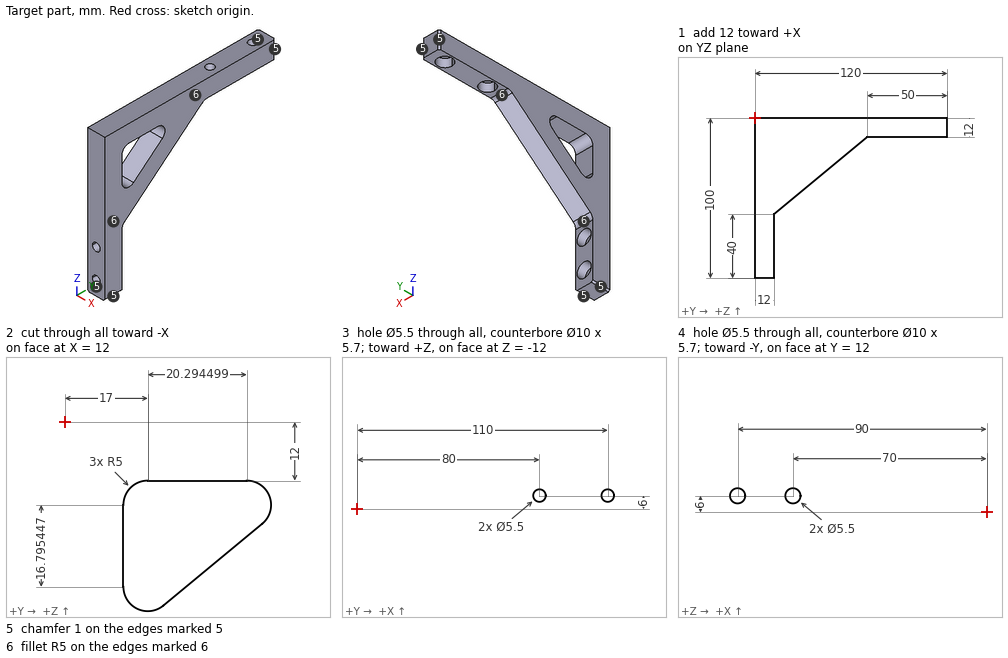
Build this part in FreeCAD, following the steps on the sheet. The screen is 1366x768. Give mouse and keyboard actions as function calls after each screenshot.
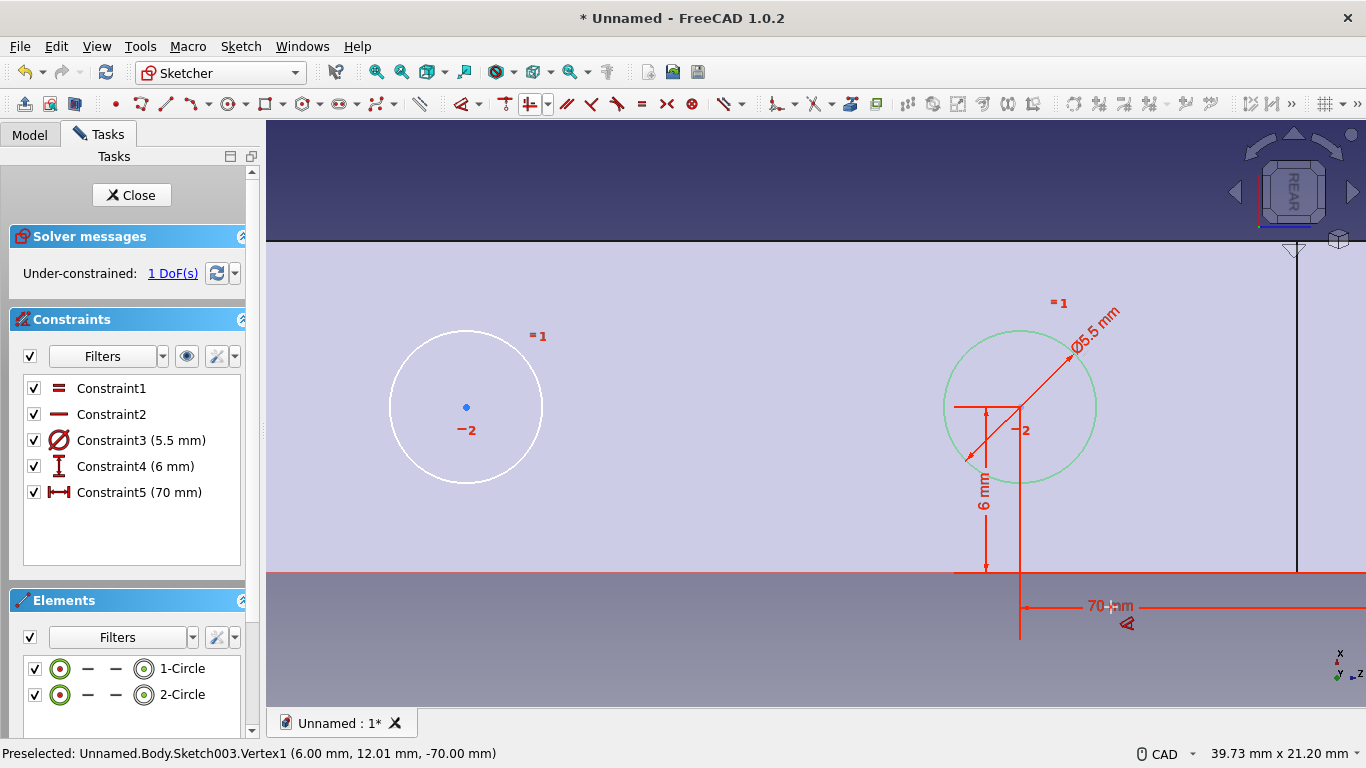
click(466, 407)
click(834, 607)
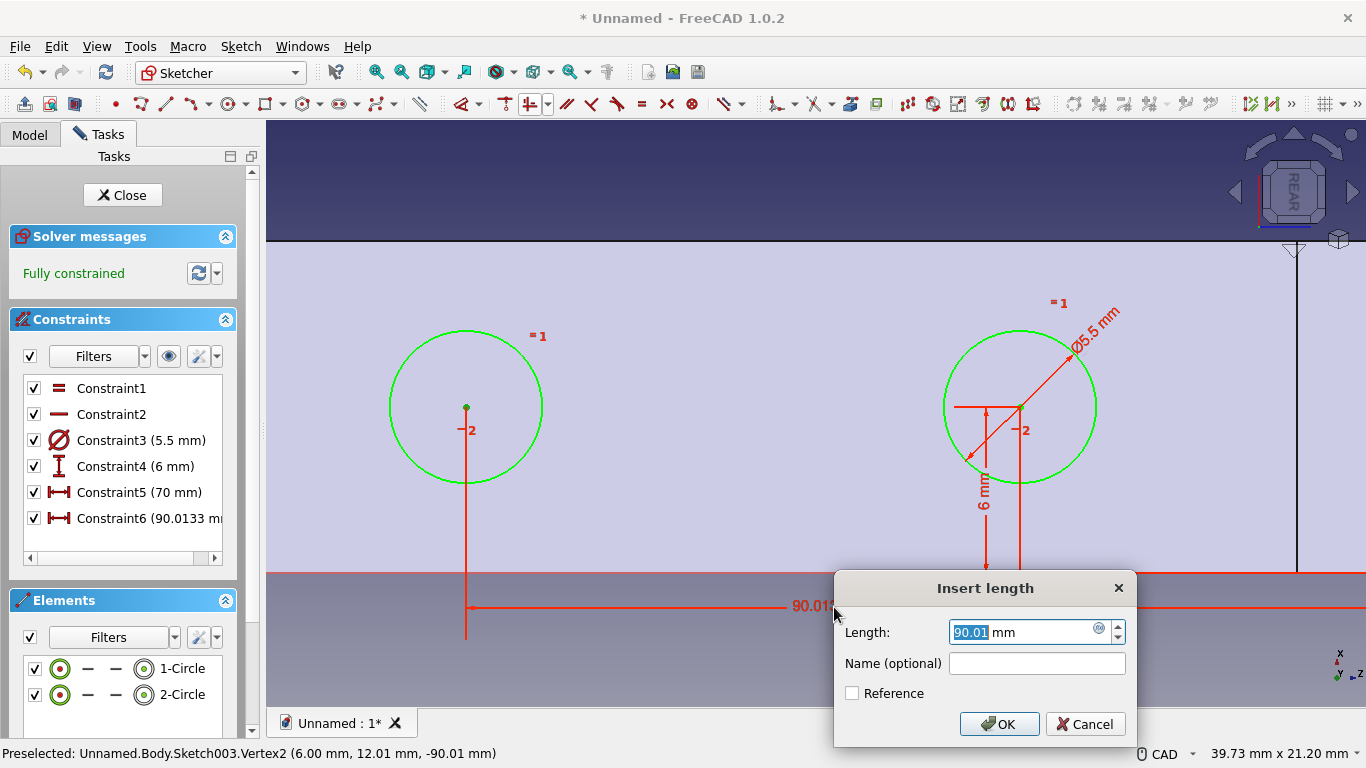
text(90)
key(Return)
key(Escape)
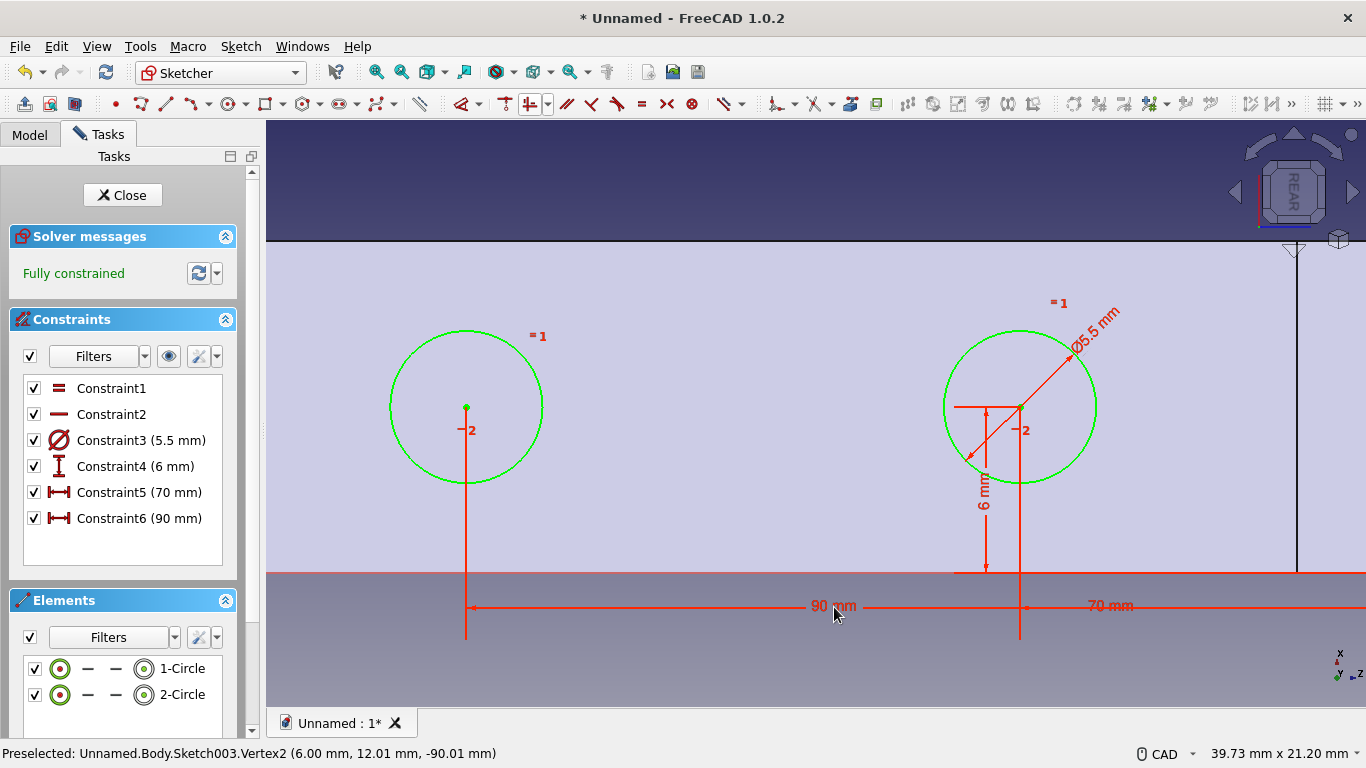
click(123, 195)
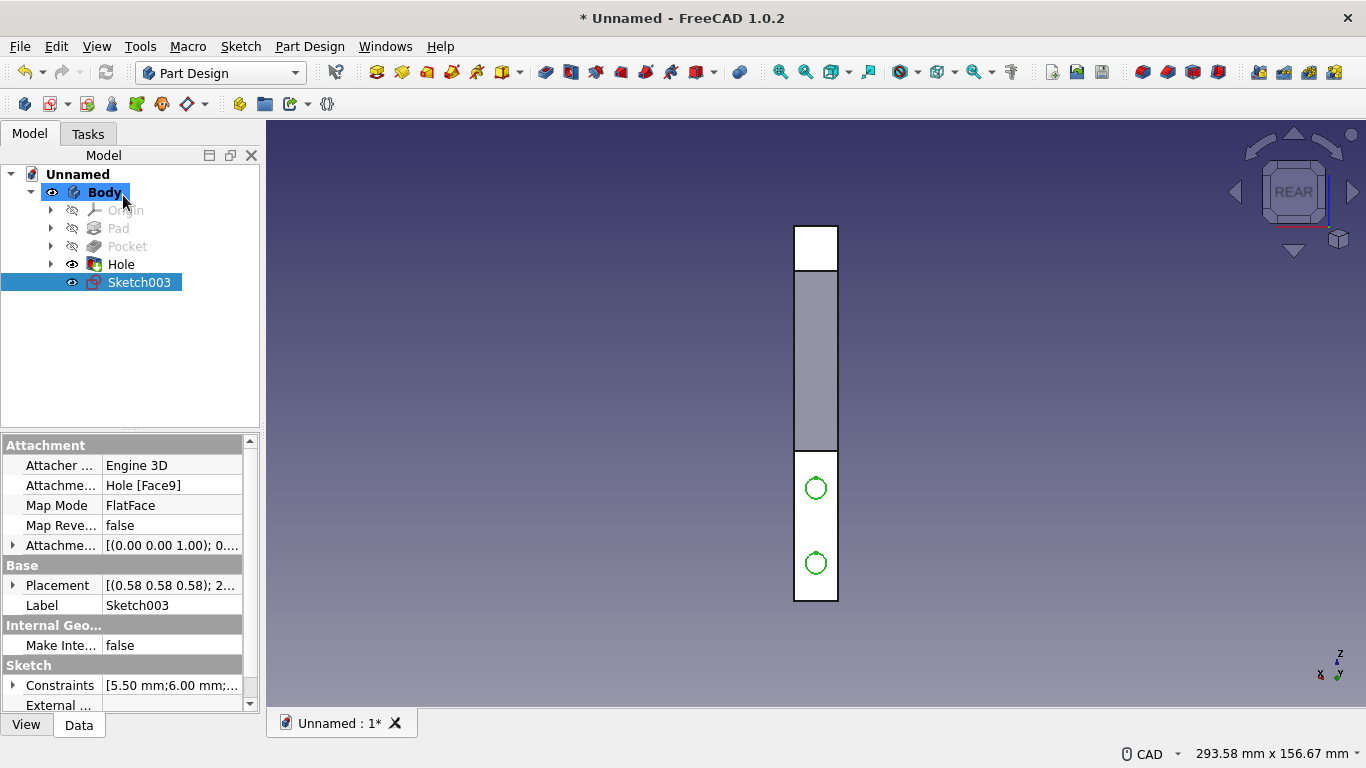
click(571, 72)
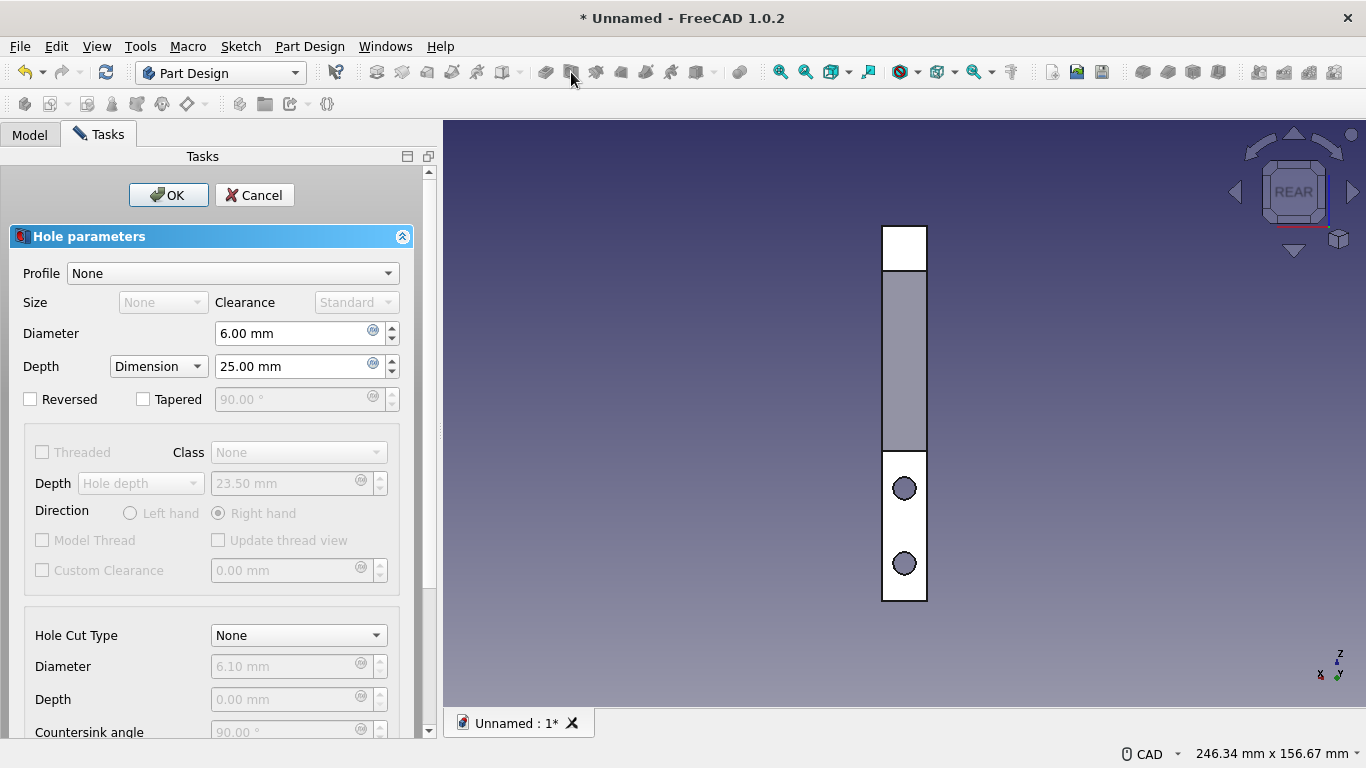
triple_click(300, 334)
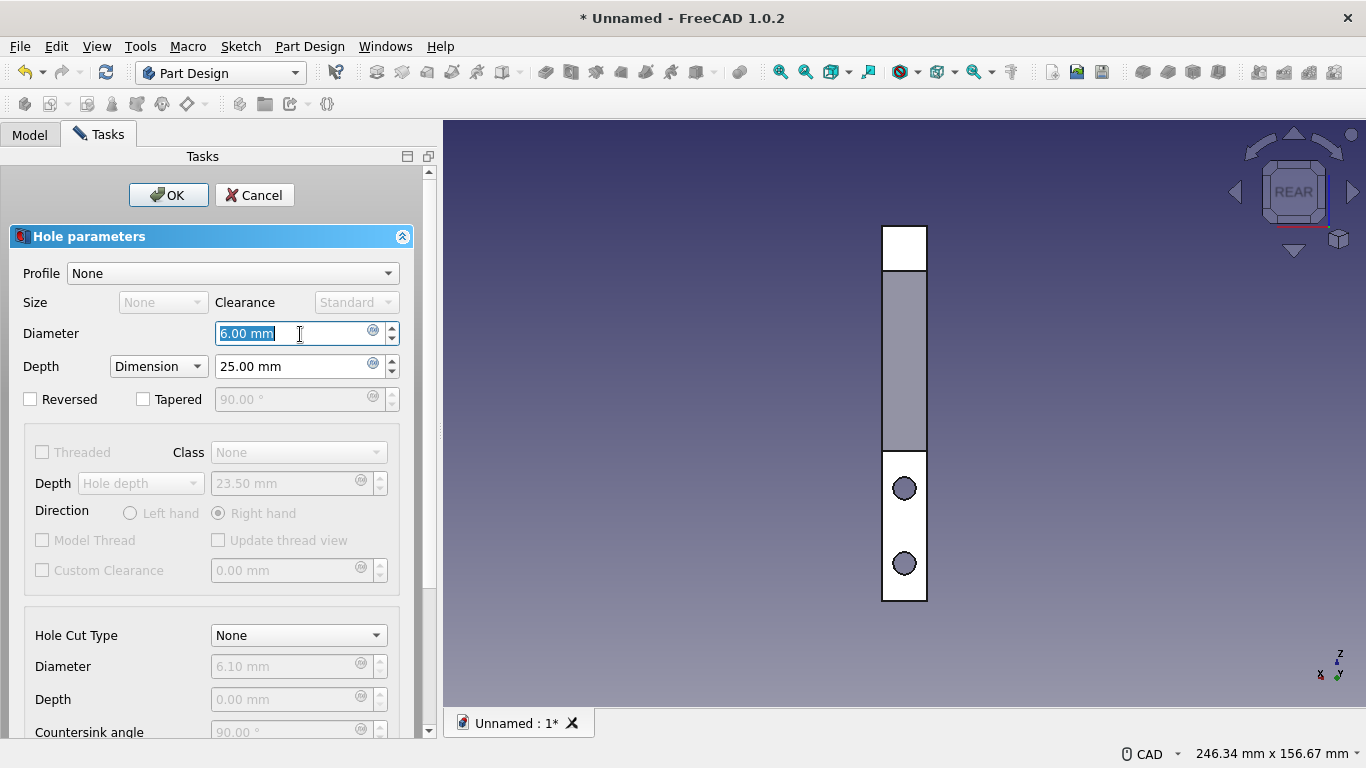
text(5.5)
key(Tab)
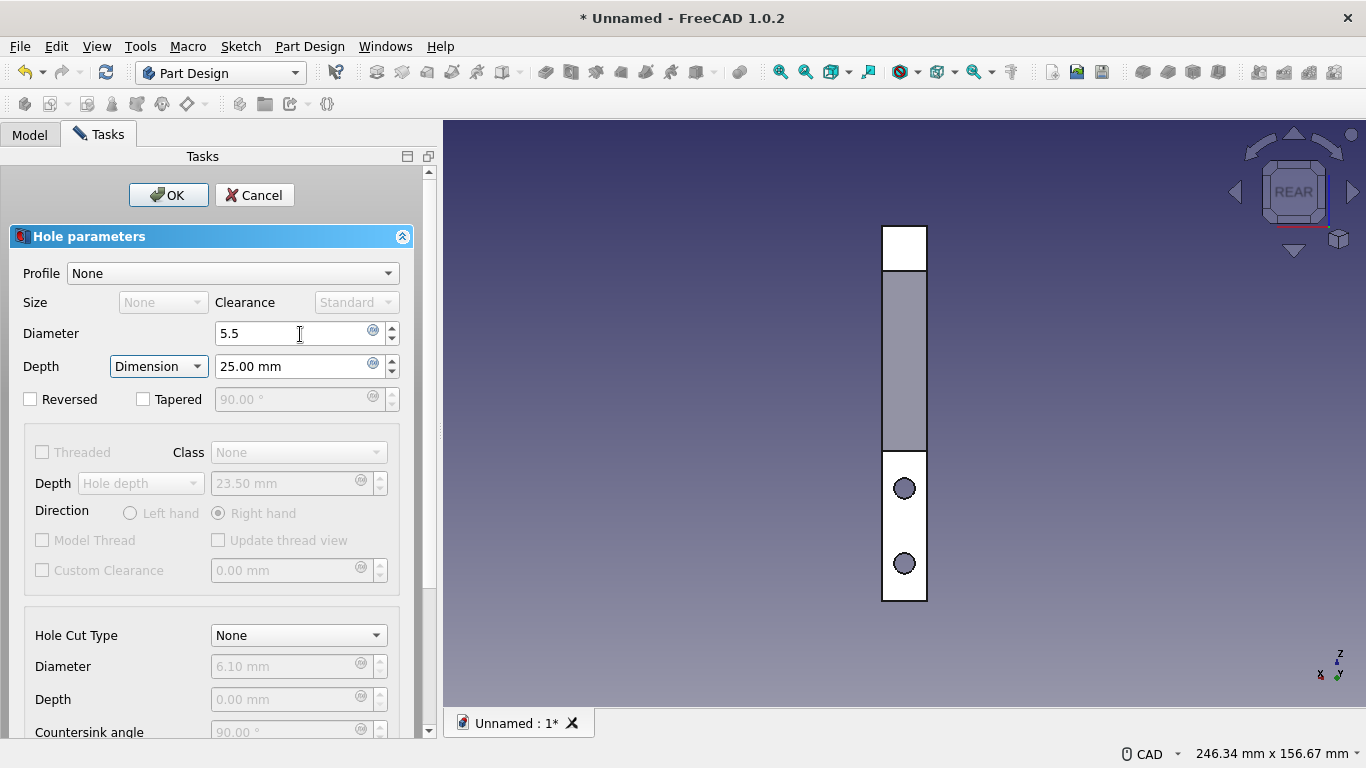
click(160, 366)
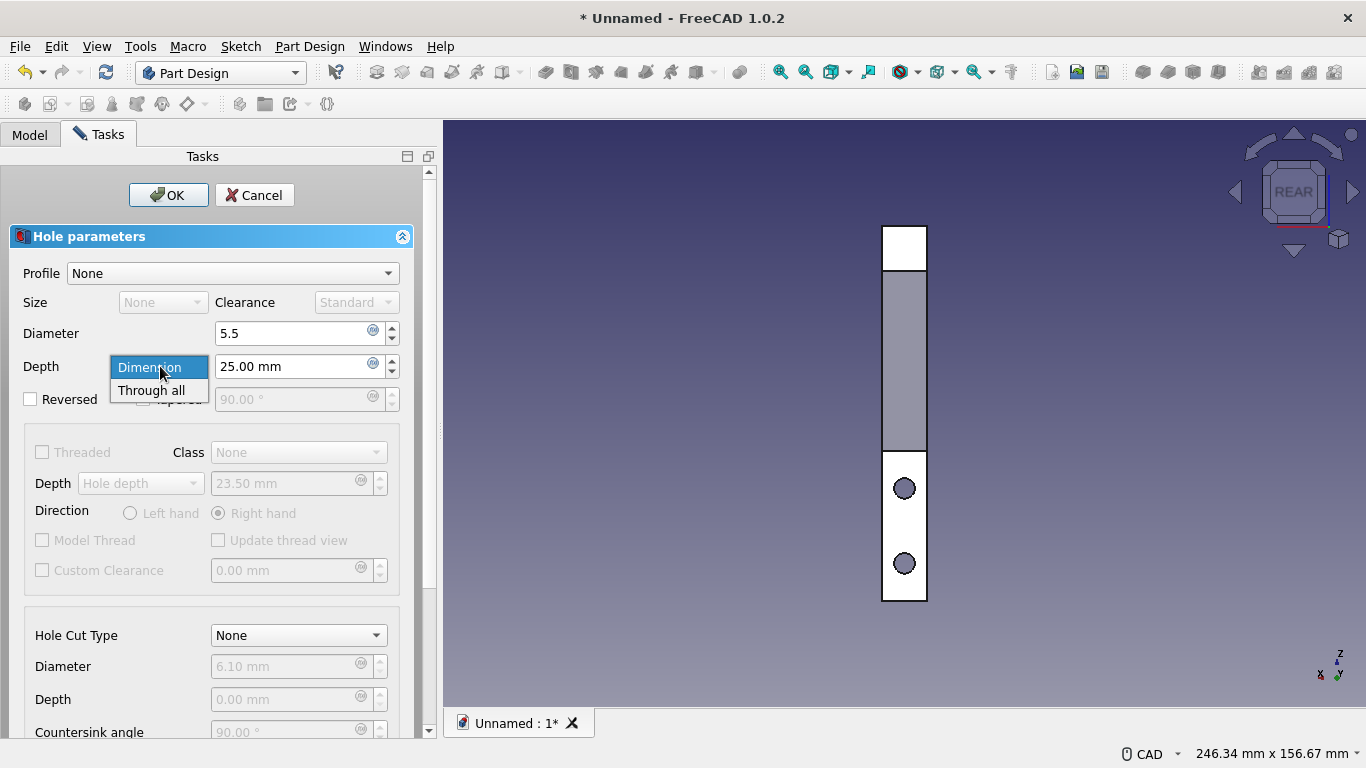
click(158, 390)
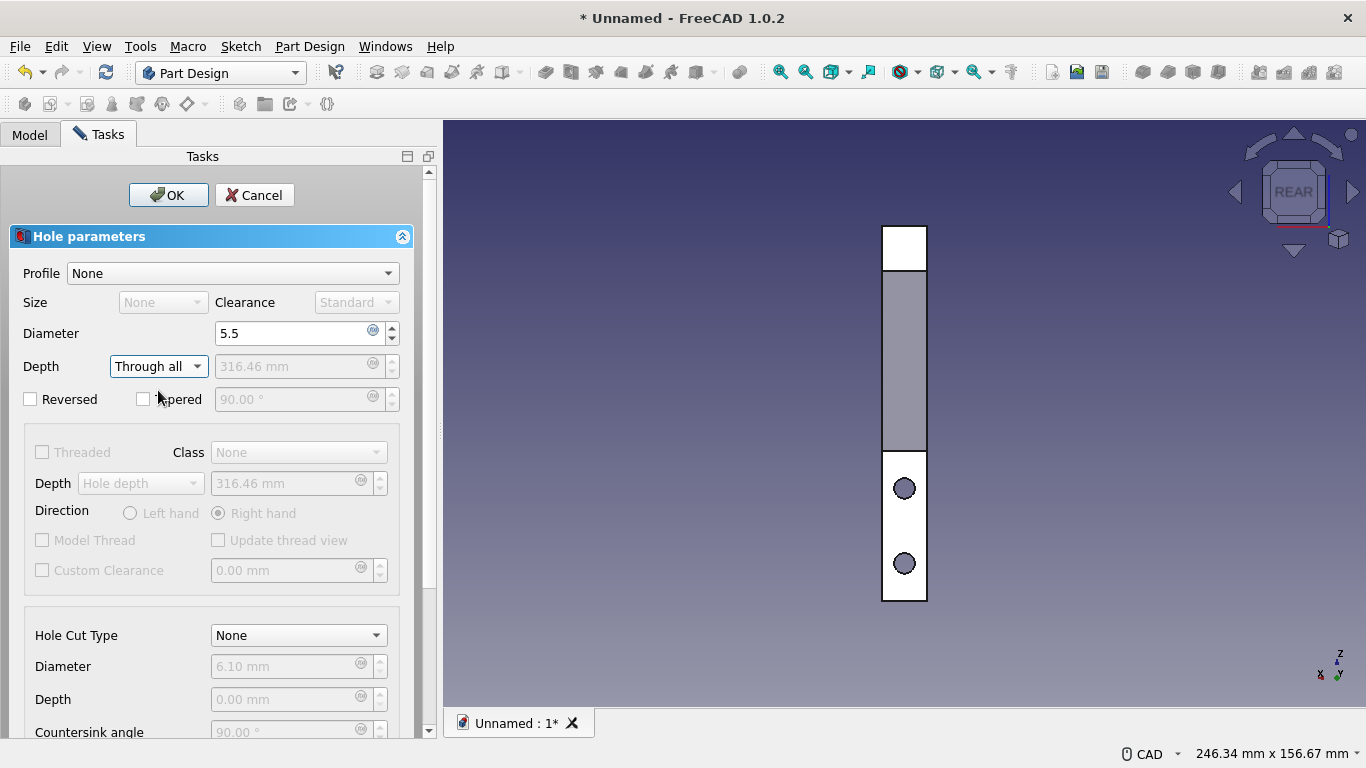
click(300, 636)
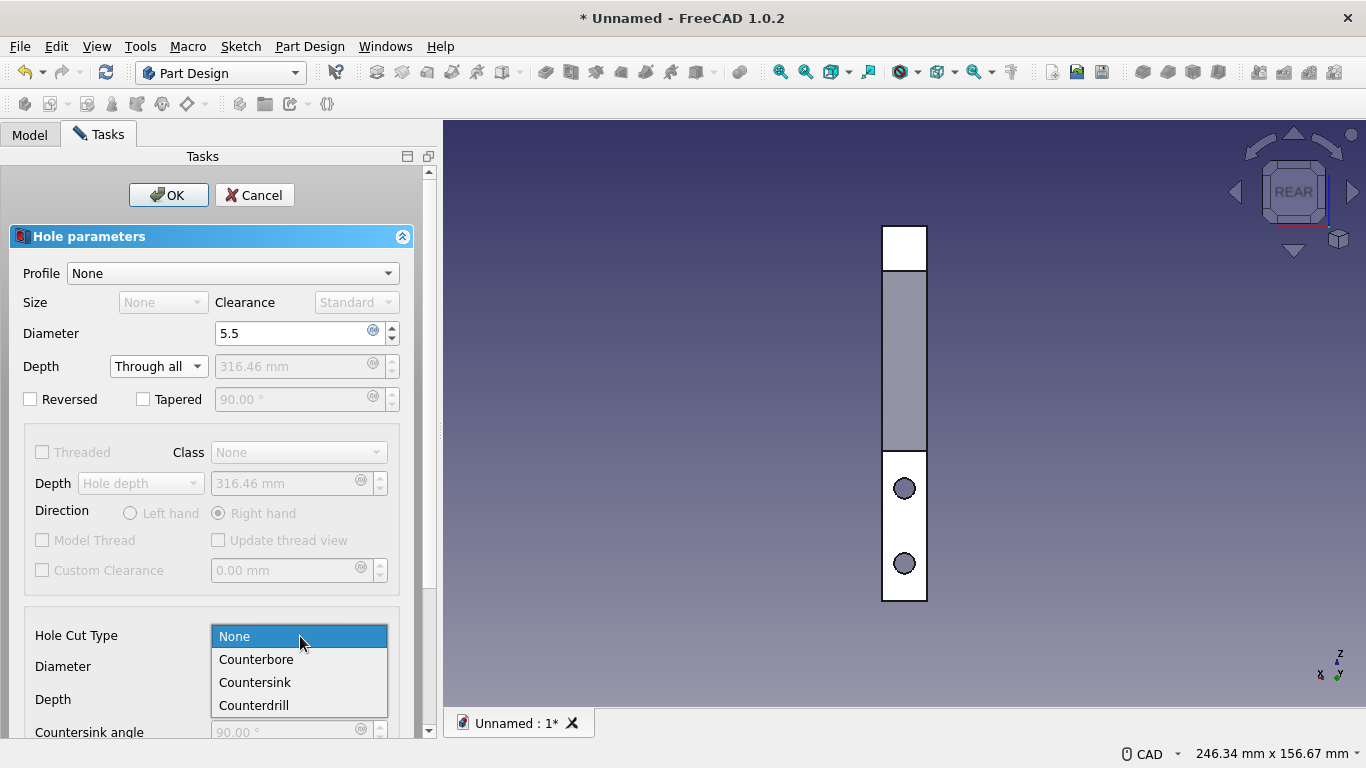
click(298, 660)